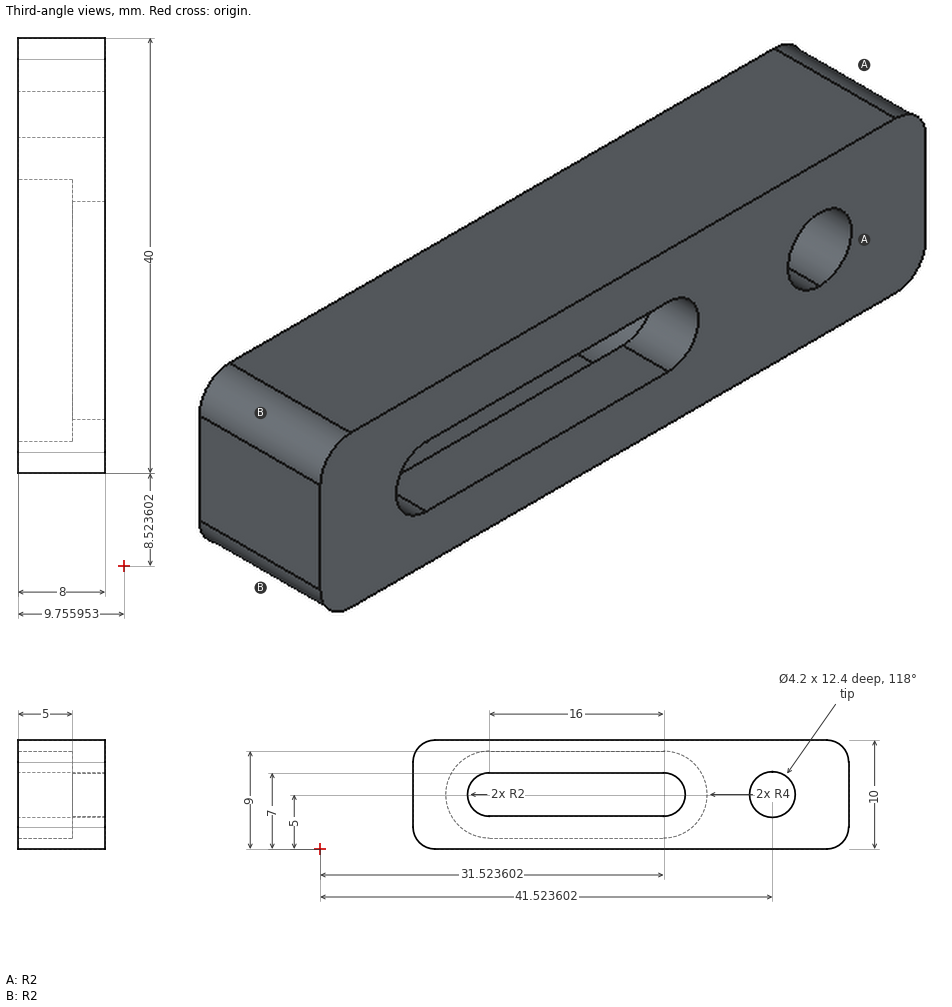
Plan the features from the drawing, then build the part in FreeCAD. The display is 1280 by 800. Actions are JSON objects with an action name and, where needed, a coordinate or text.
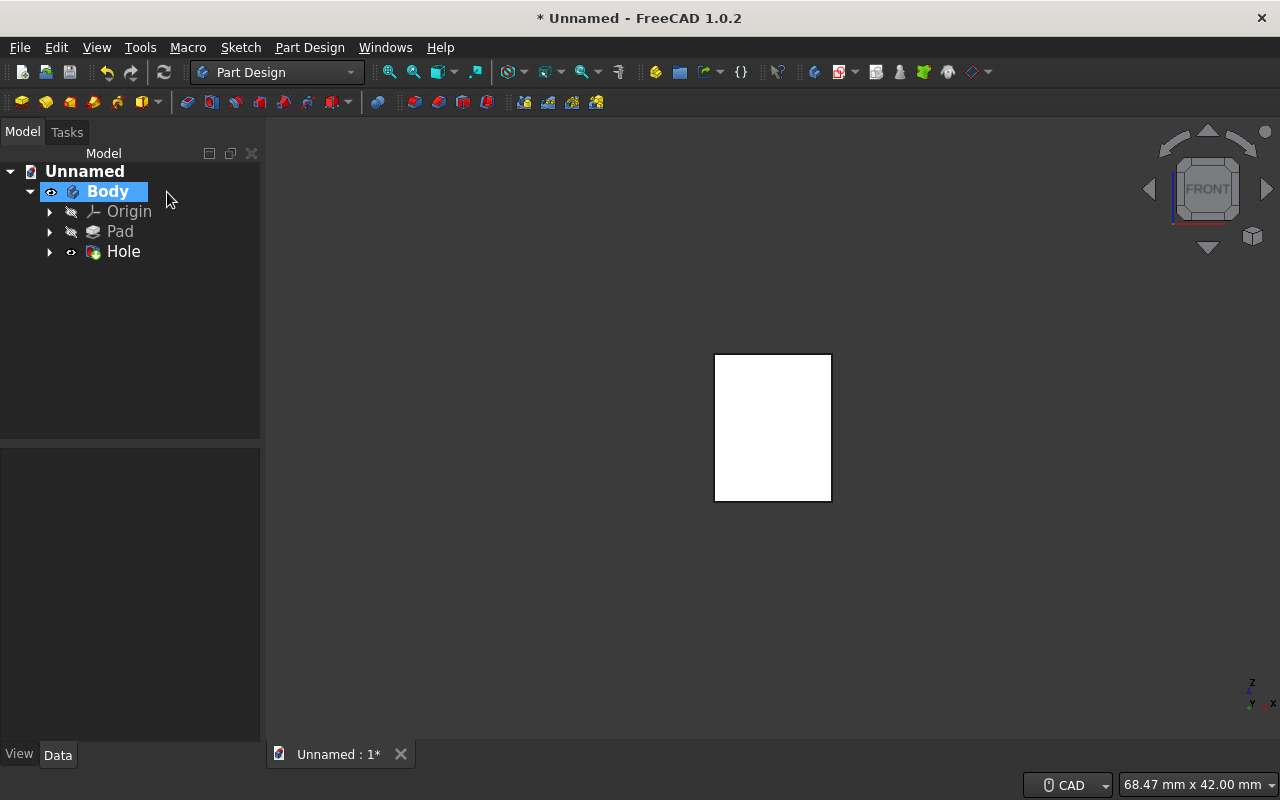
{"action": "key", "text": "v f"}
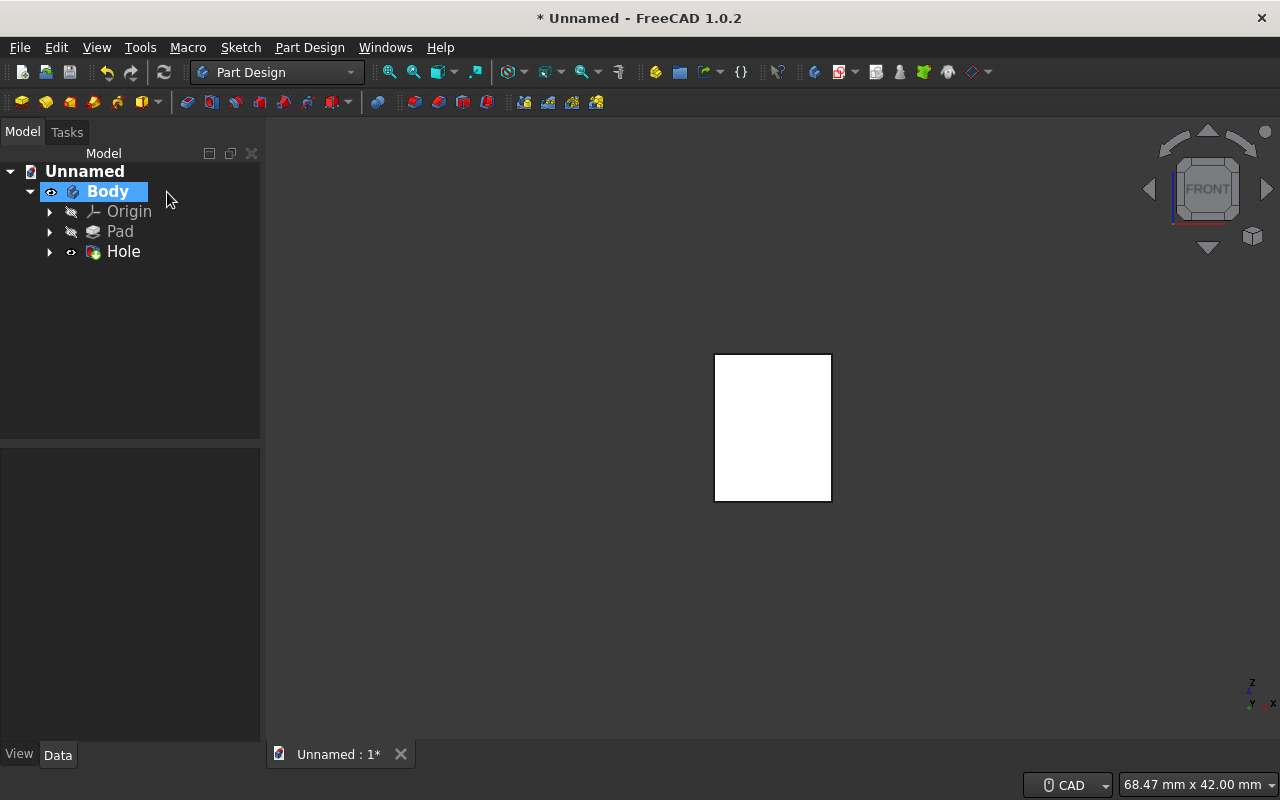
{"action": "key", "text": "3"}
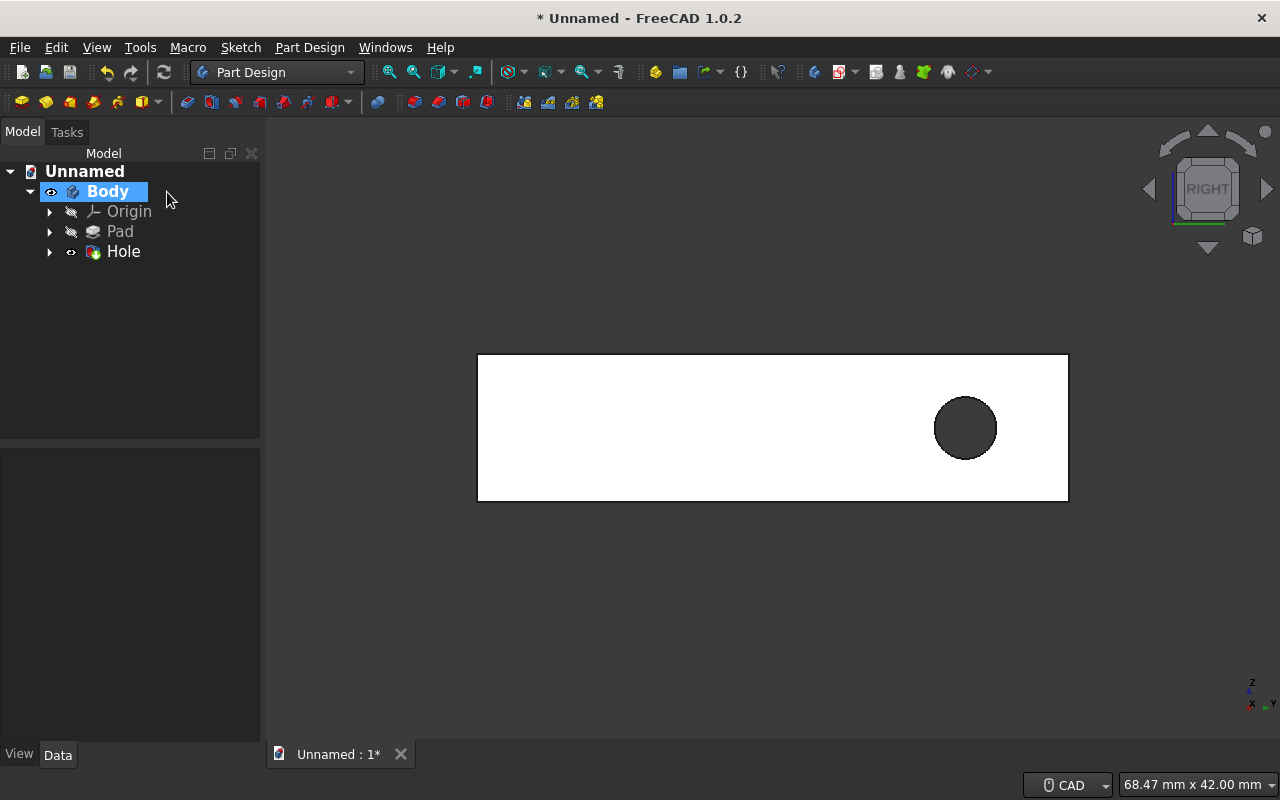
{"action": "key", "text": "5"}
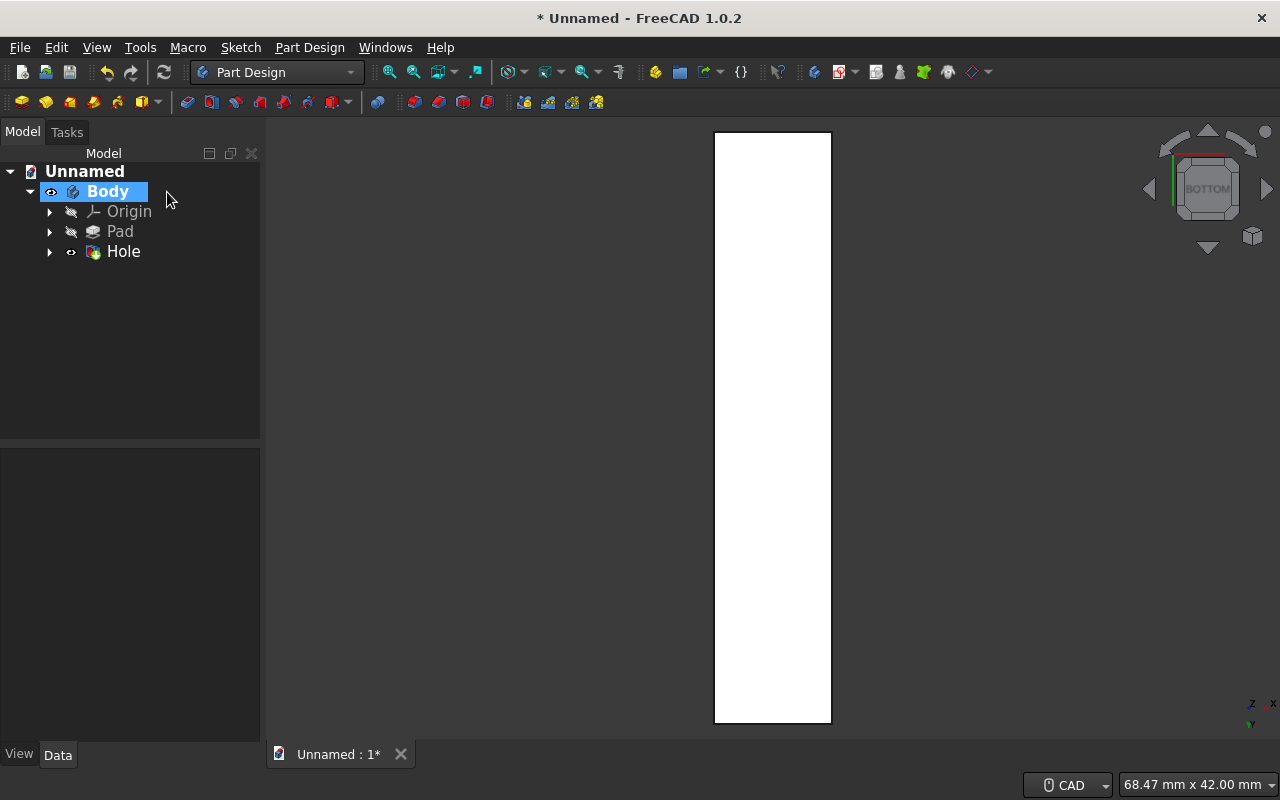
{"action": "key", "text": "4"}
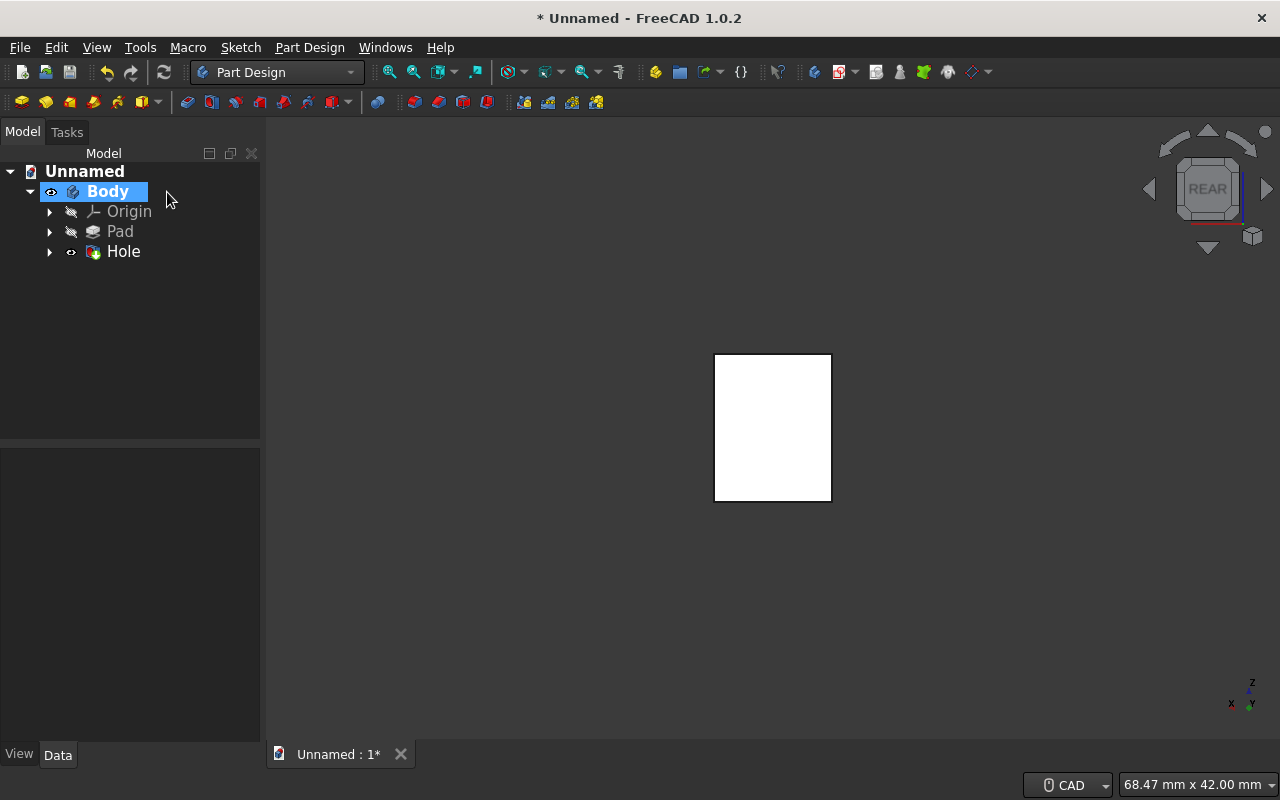
{"action": "left_click", "coordinate": [390, 72]}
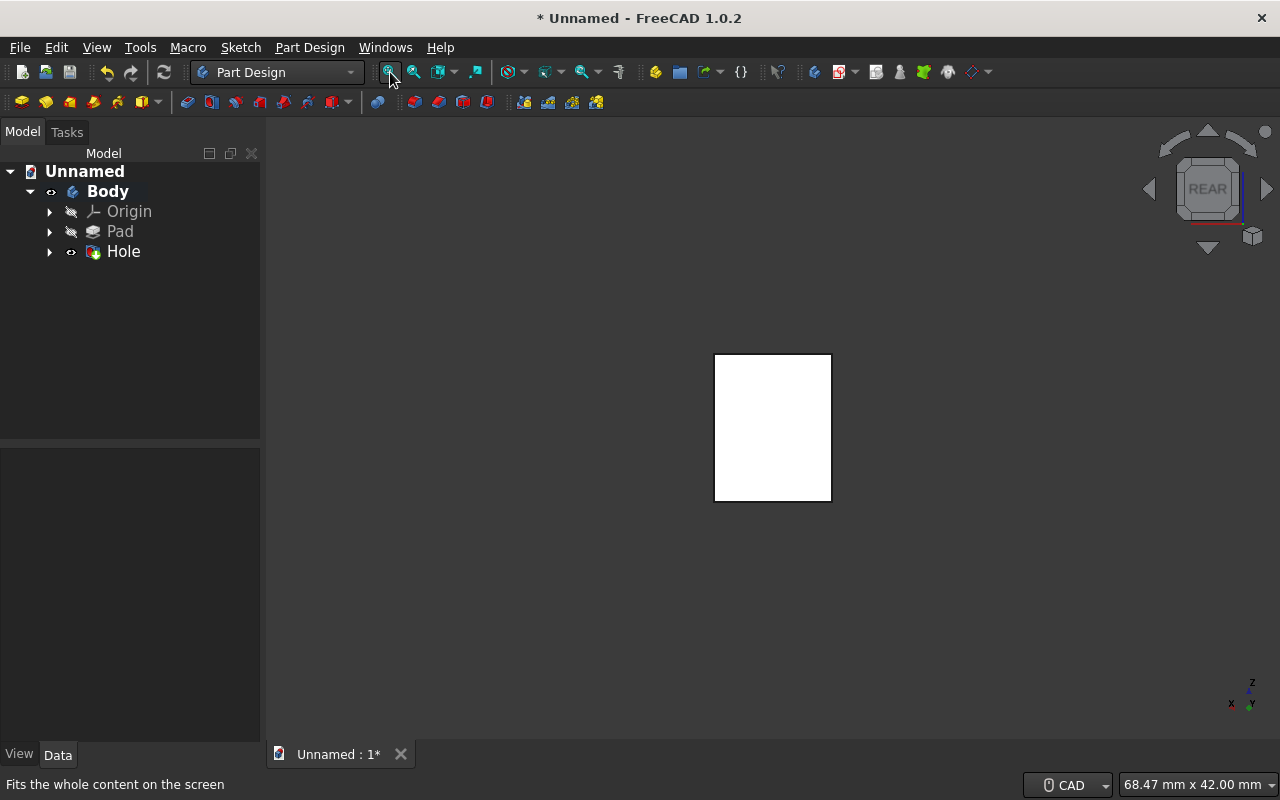
{"action": "left_click", "coordinate": [773, 353]}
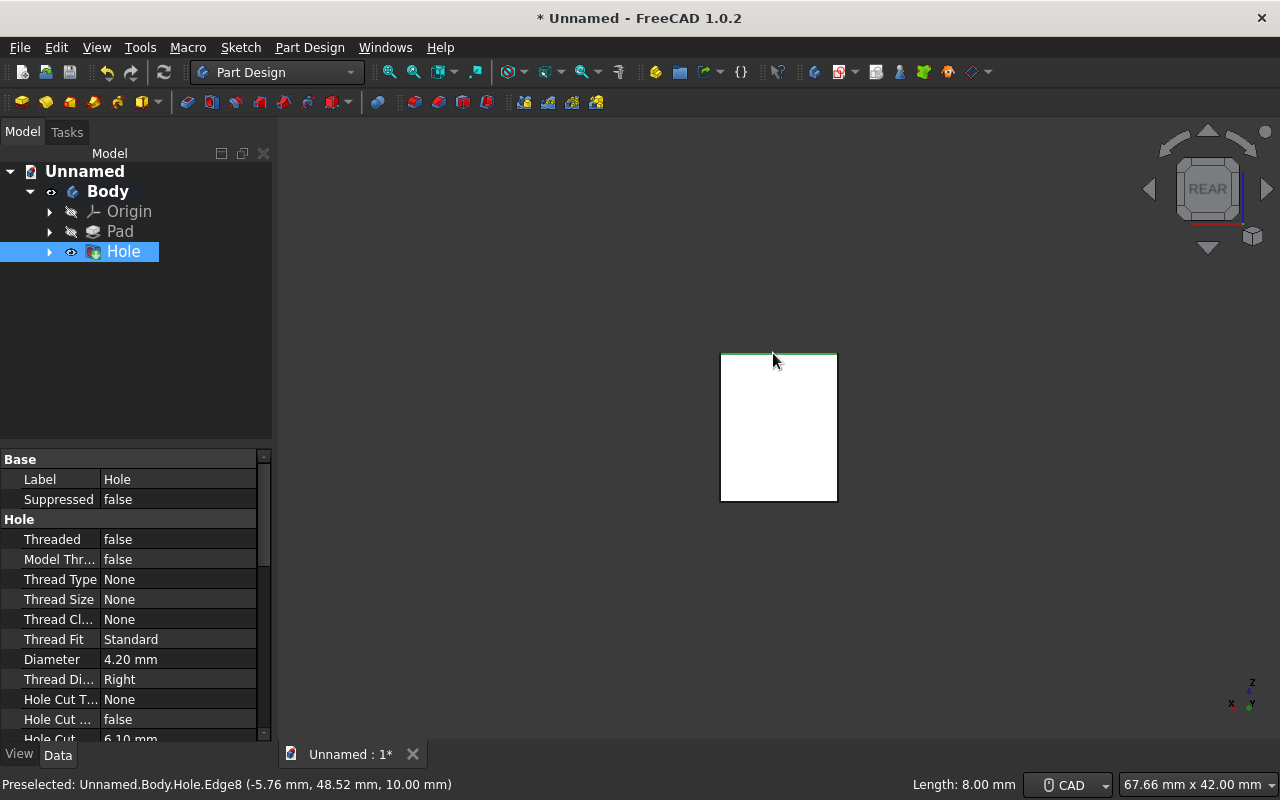
{"action": "left_click", "coordinate": [779, 501], "text": "ctrl"}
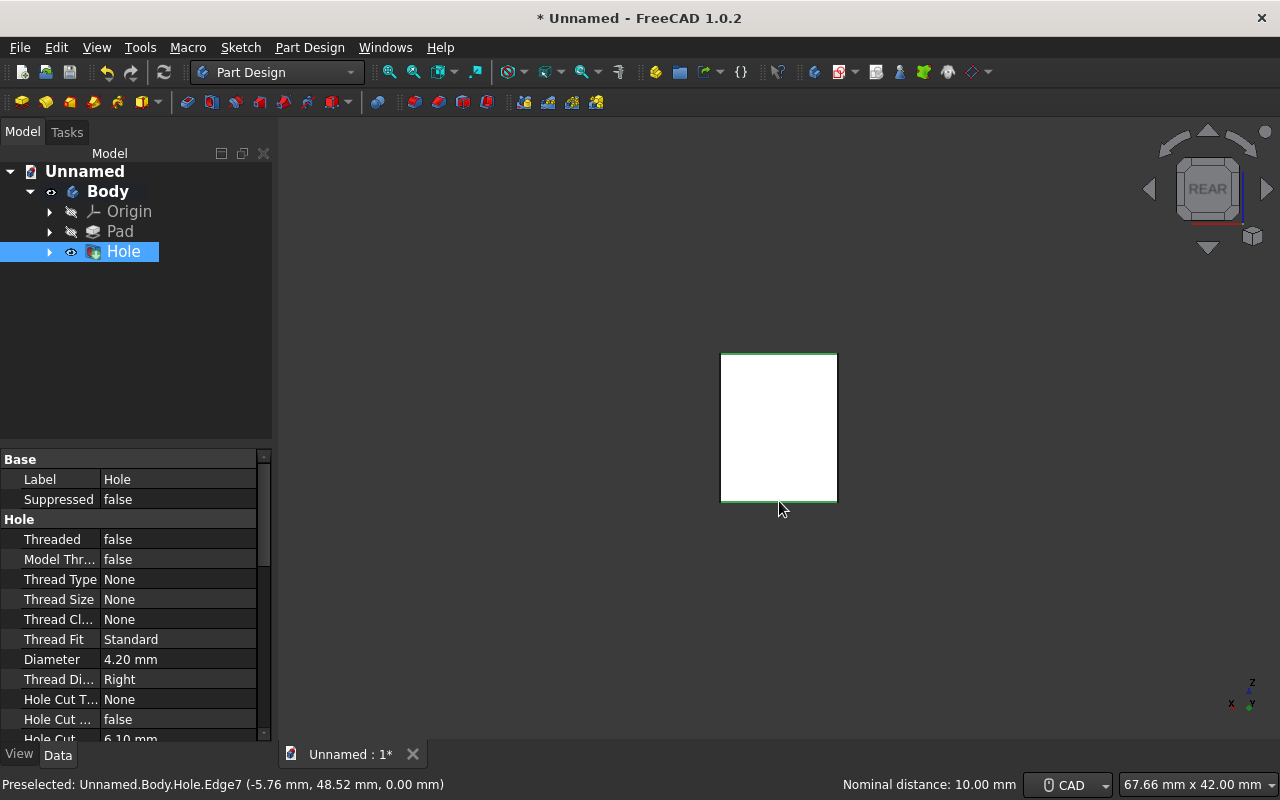
{"action": "left_click", "coordinate": [416, 102]}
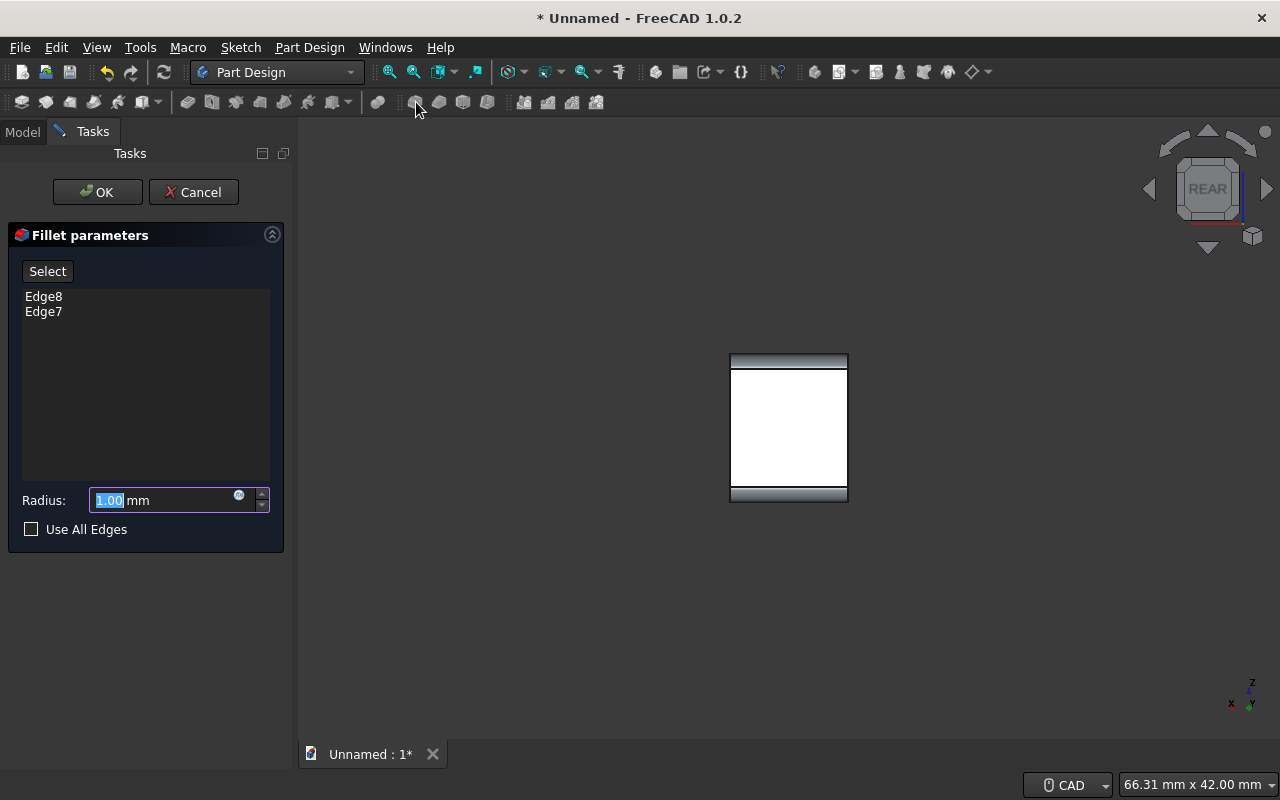
{"action": "type", "text": "2"}
{"action": "key", "text": "Tab"}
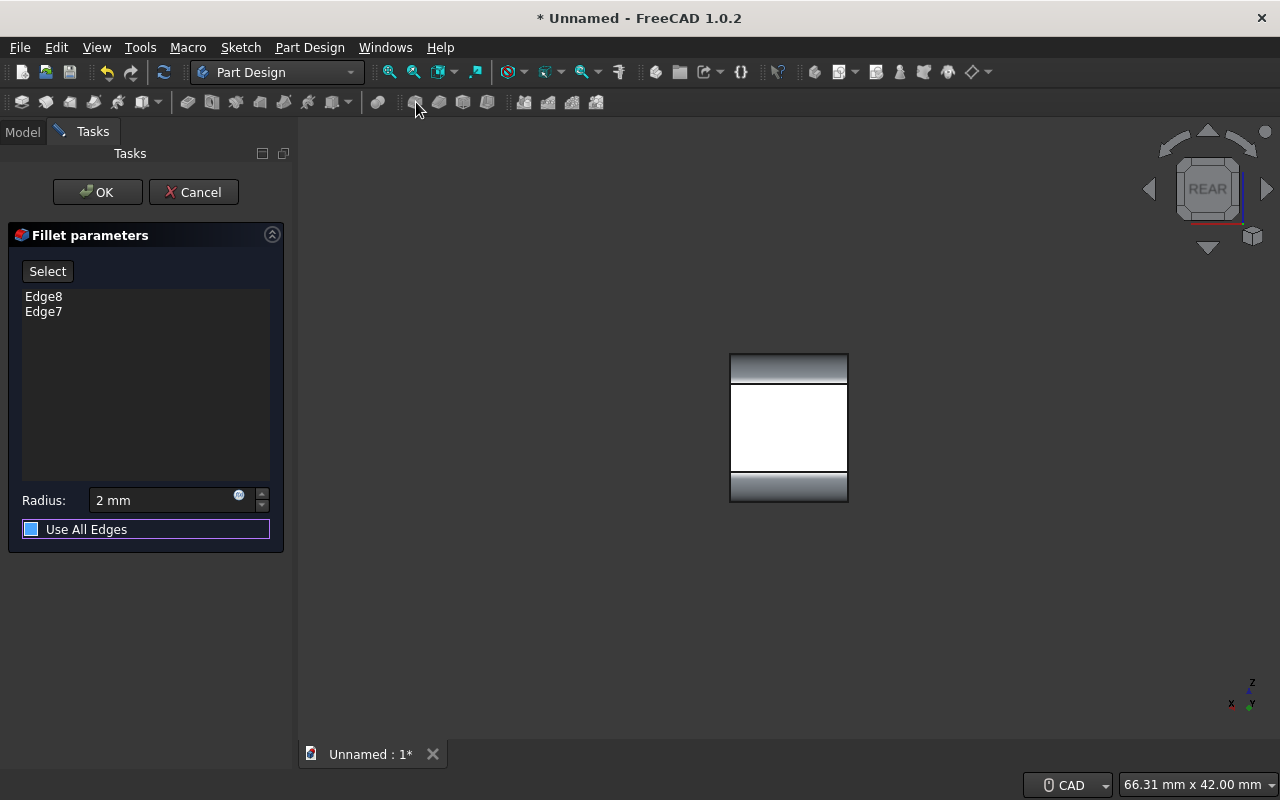
{"action": "left_click", "coordinate": [98, 192]}